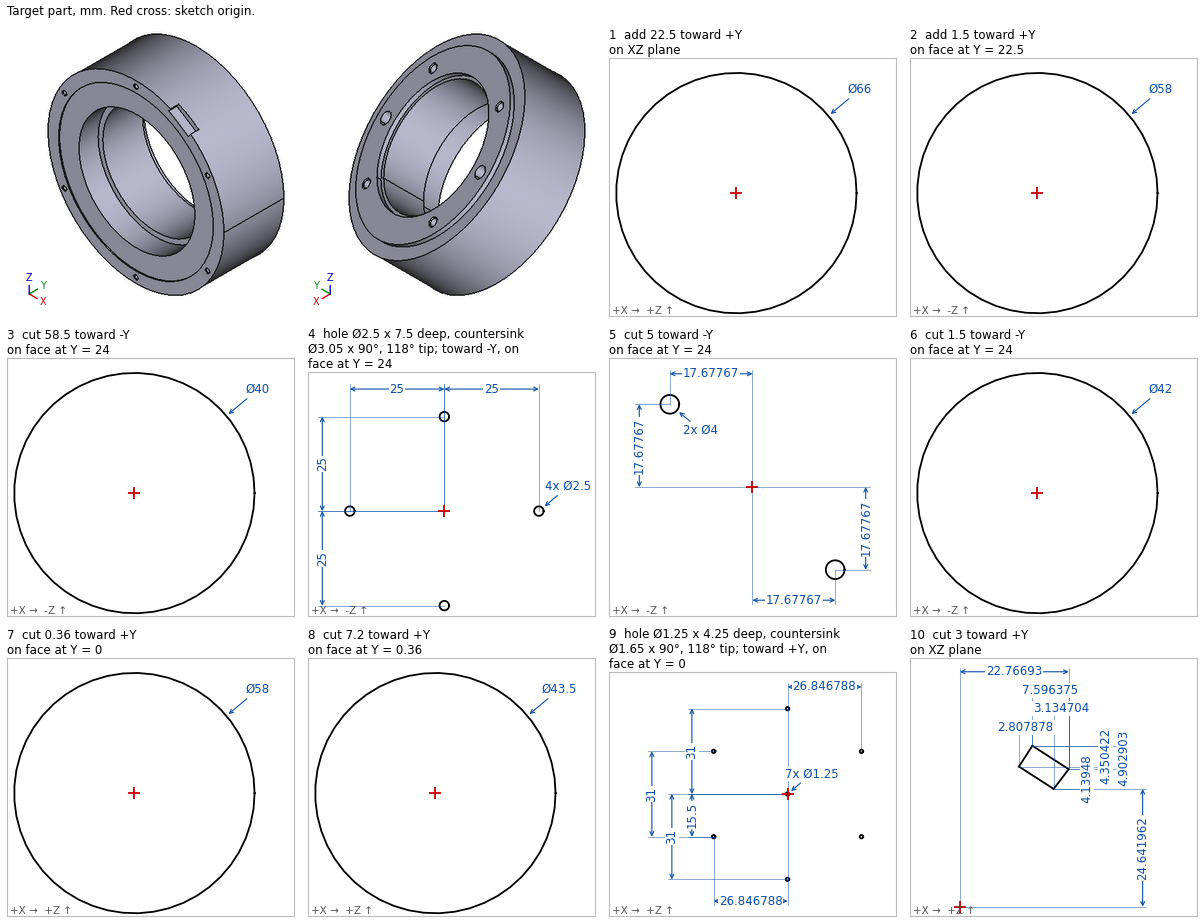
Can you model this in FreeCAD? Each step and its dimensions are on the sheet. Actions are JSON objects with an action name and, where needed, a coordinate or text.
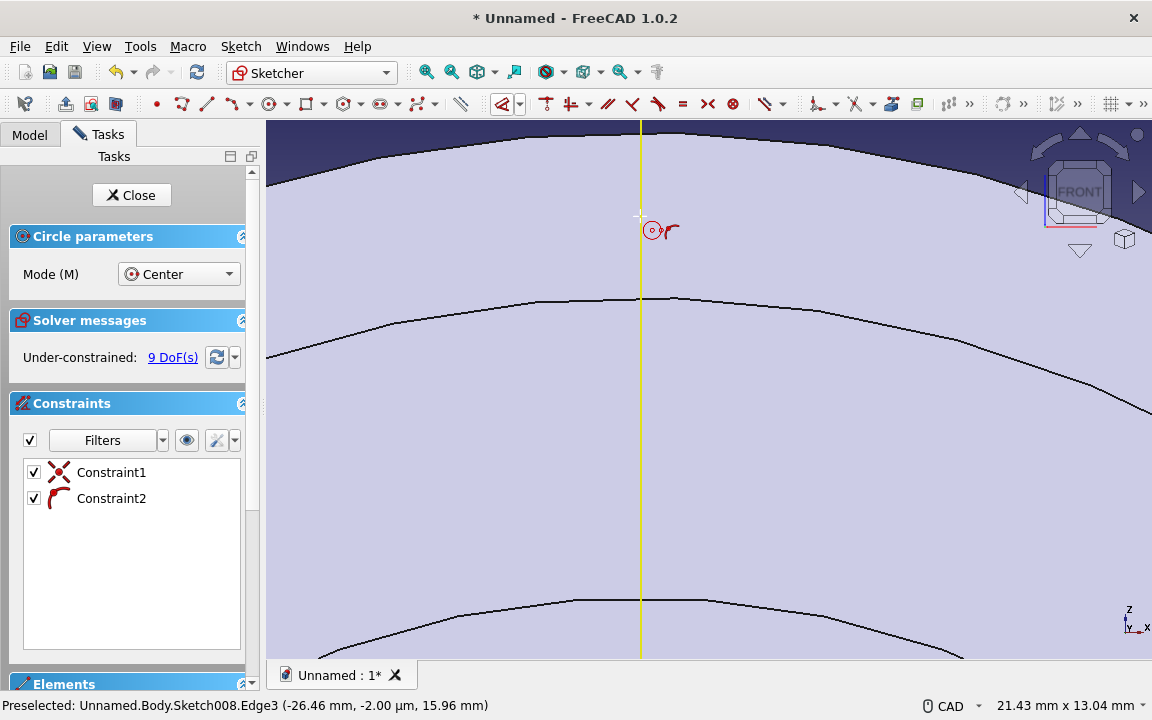
{"action": "scroll", "coordinate": [640, 216], "scroll_direction": "down", "scroll_amount": 10}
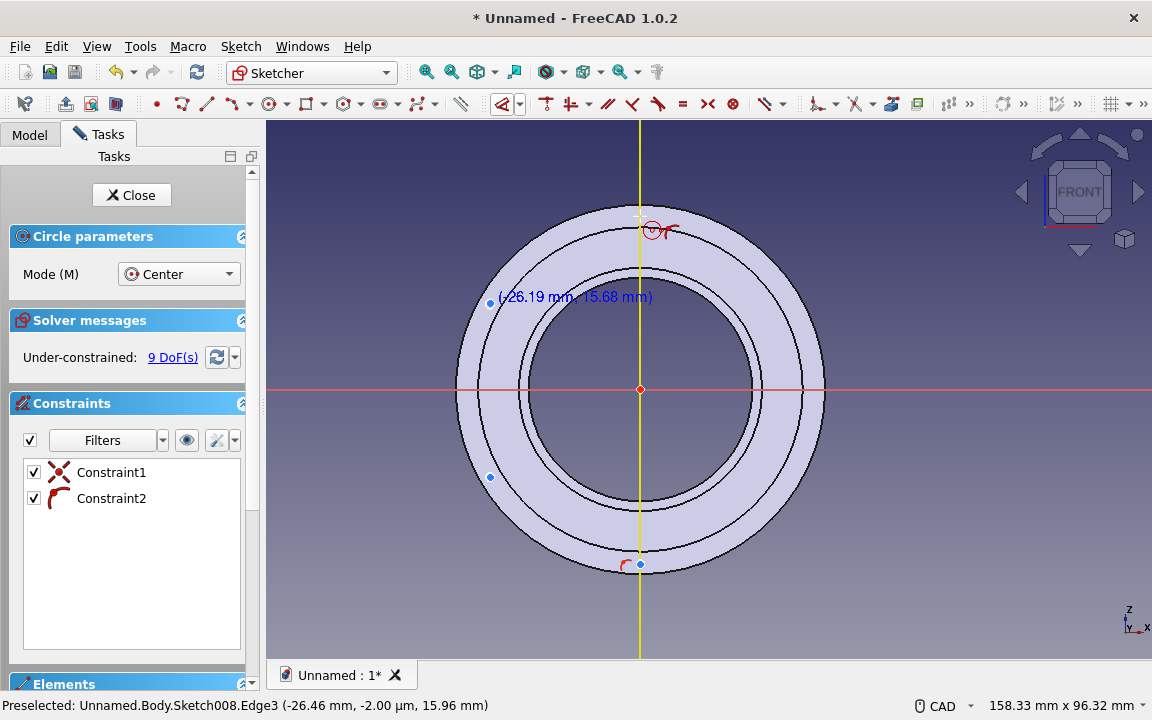
{"action": "left_click", "coordinate": [640, 216]}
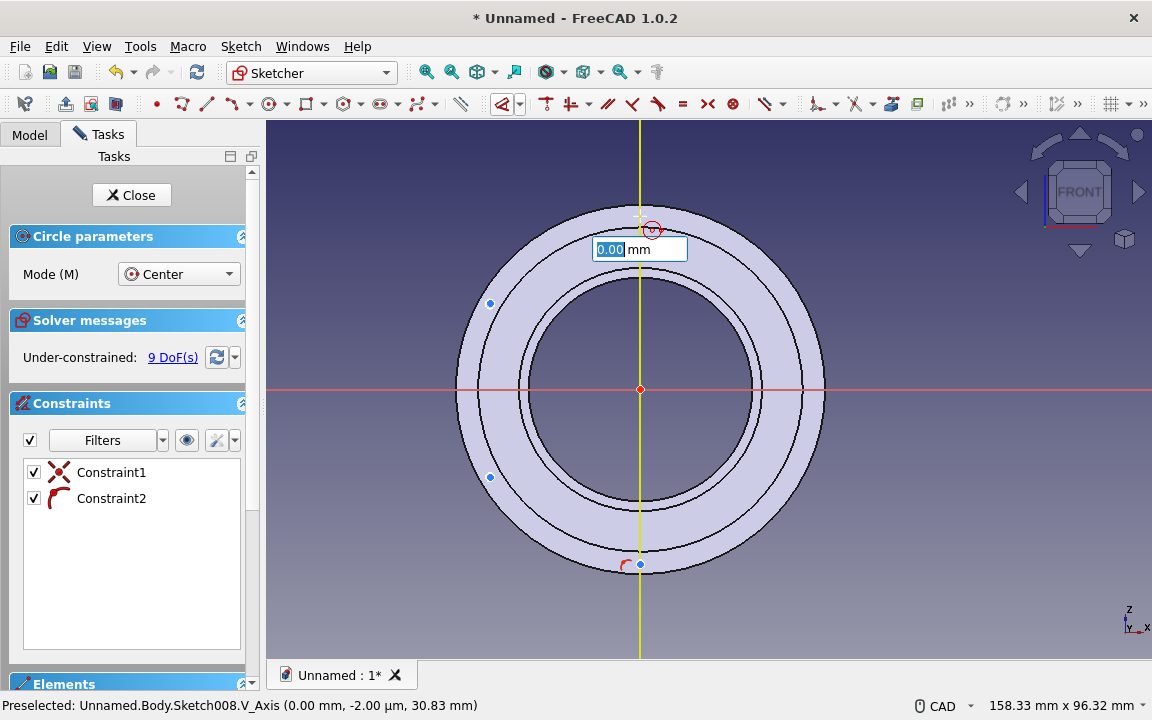
{"action": "scroll", "coordinate": [644, 215], "scroll_direction": "up", "scroll_amount": 8}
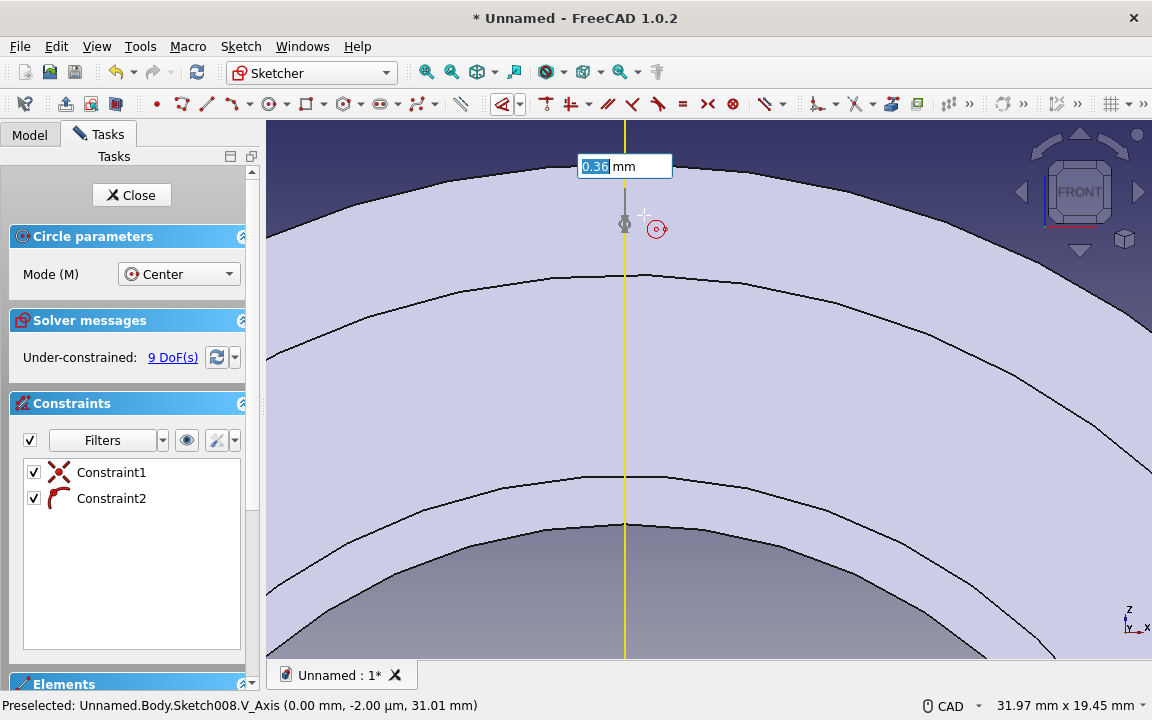
{"action": "left_click", "coordinate": [641, 213]}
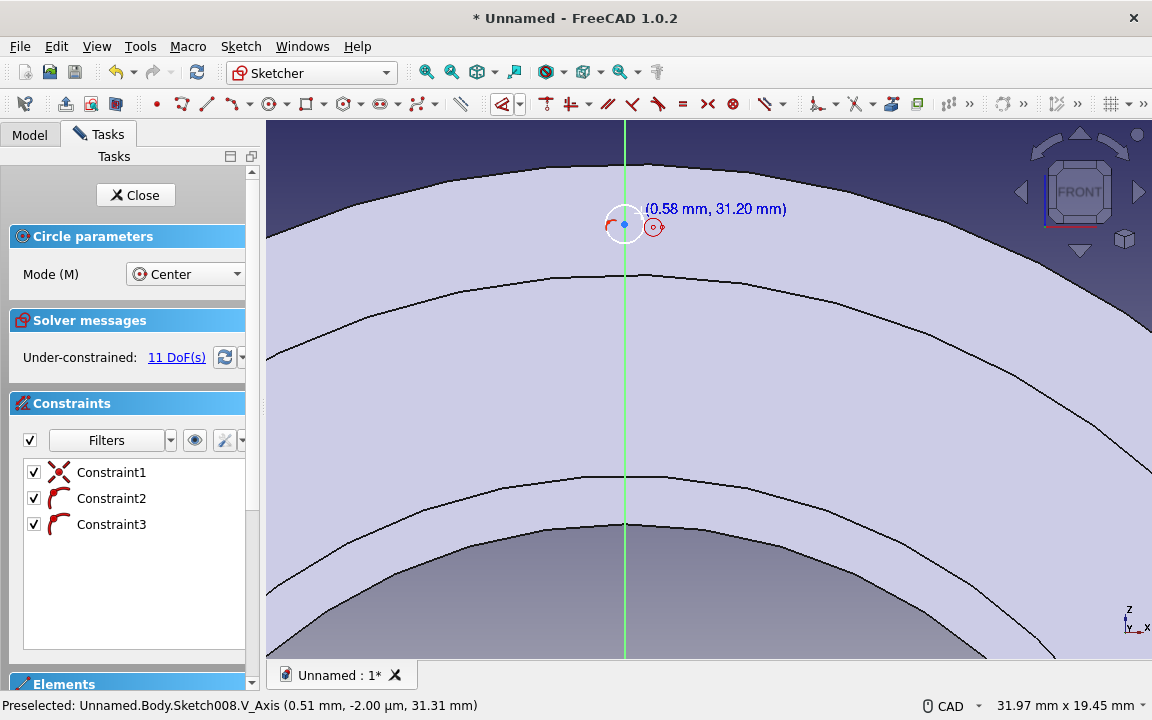
{"action": "scroll", "coordinate": [644, 215], "scroll_direction": "down", "scroll_amount": 8}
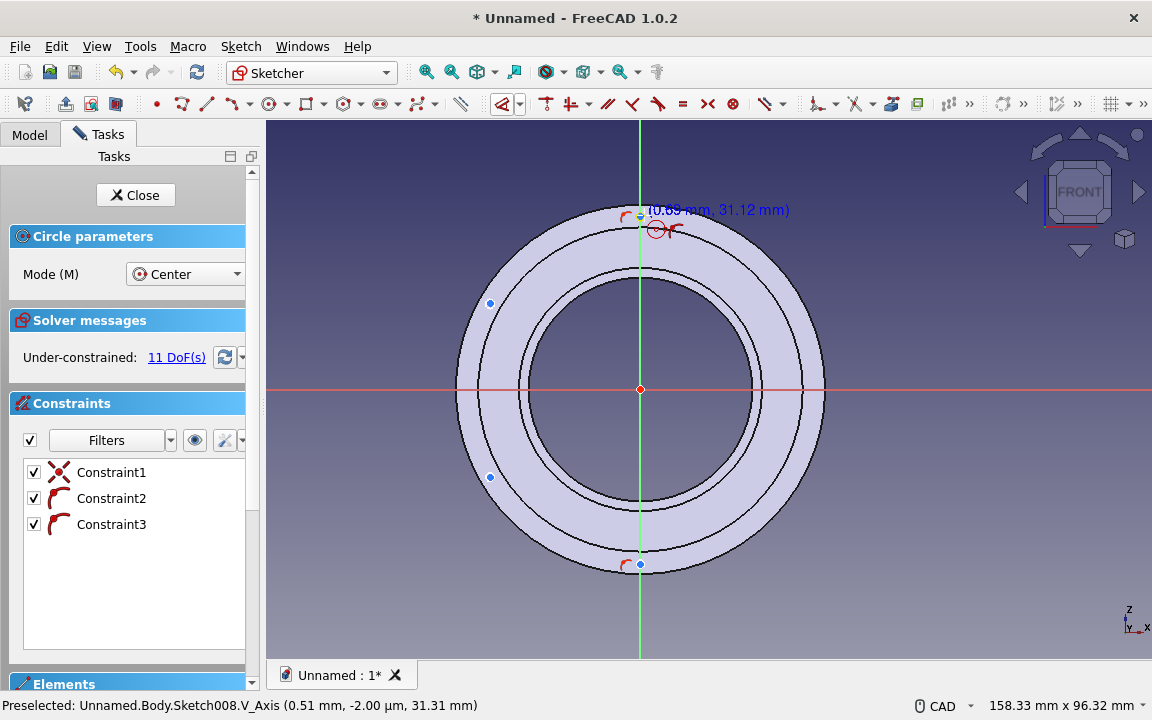
{"action": "scroll", "coordinate": [791, 303], "scroll_direction": "up", "scroll_amount": 10}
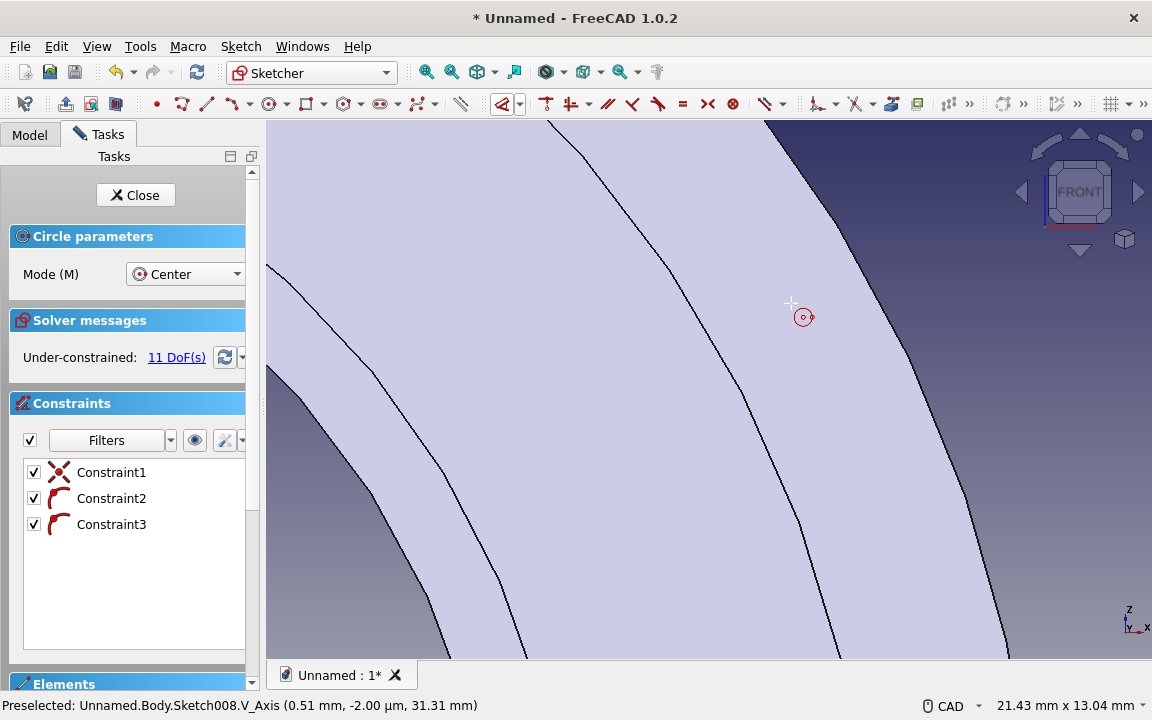
{"action": "scroll", "coordinate": [792, 303], "scroll_direction": "down", "scroll_amount": 10}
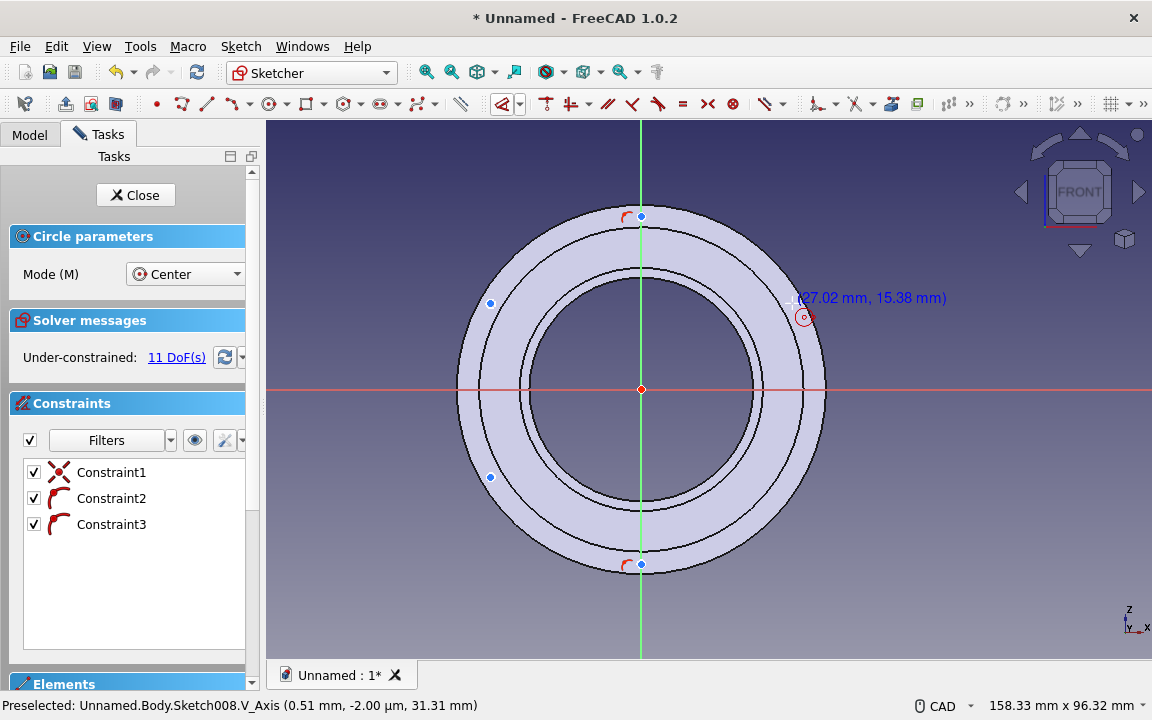
{"action": "left_click", "coordinate": [792, 303]}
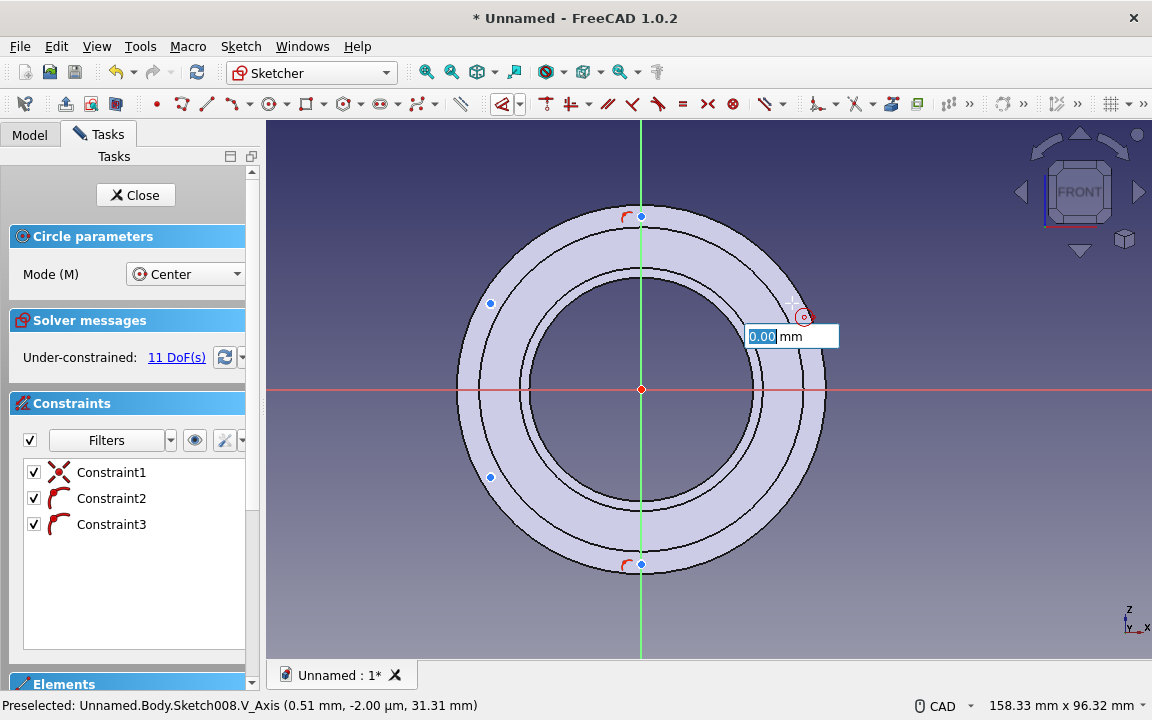
{"action": "scroll", "coordinate": [794, 300], "scroll_direction": "up", "scroll_amount": 8}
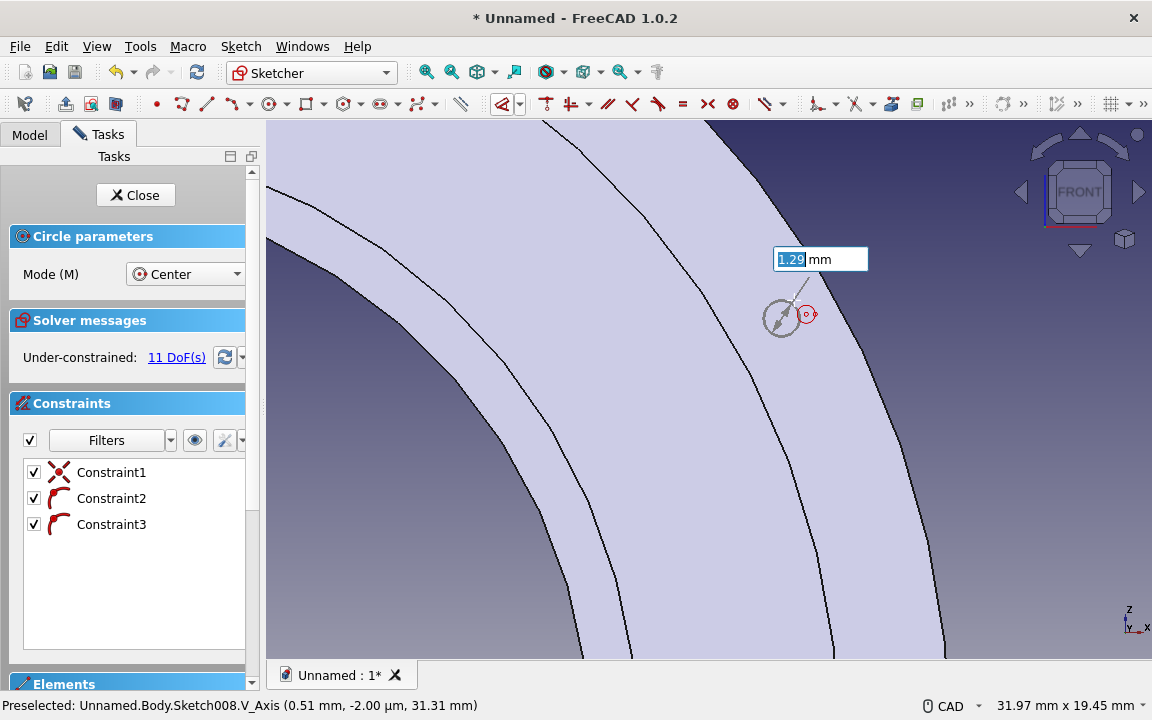
{"action": "left_click", "coordinate": [792, 300]}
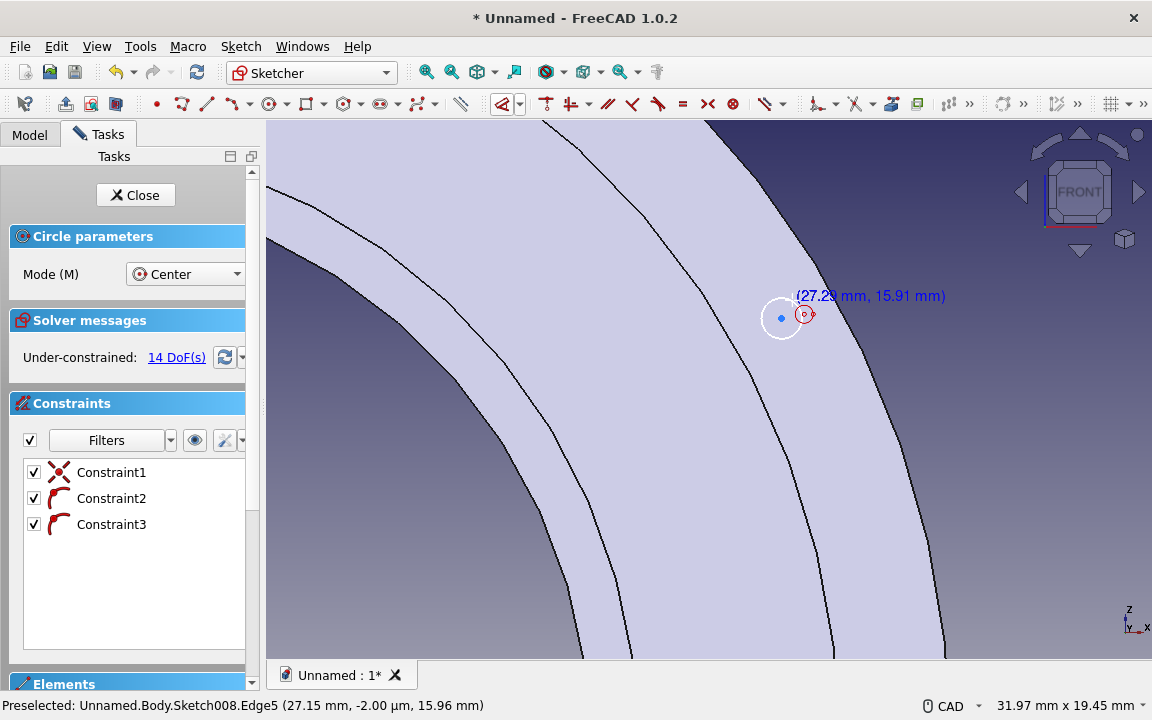
{"action": "scroll", "coordinate": [794, 300], "scroll_direction": "down", "scroll_amount": 8}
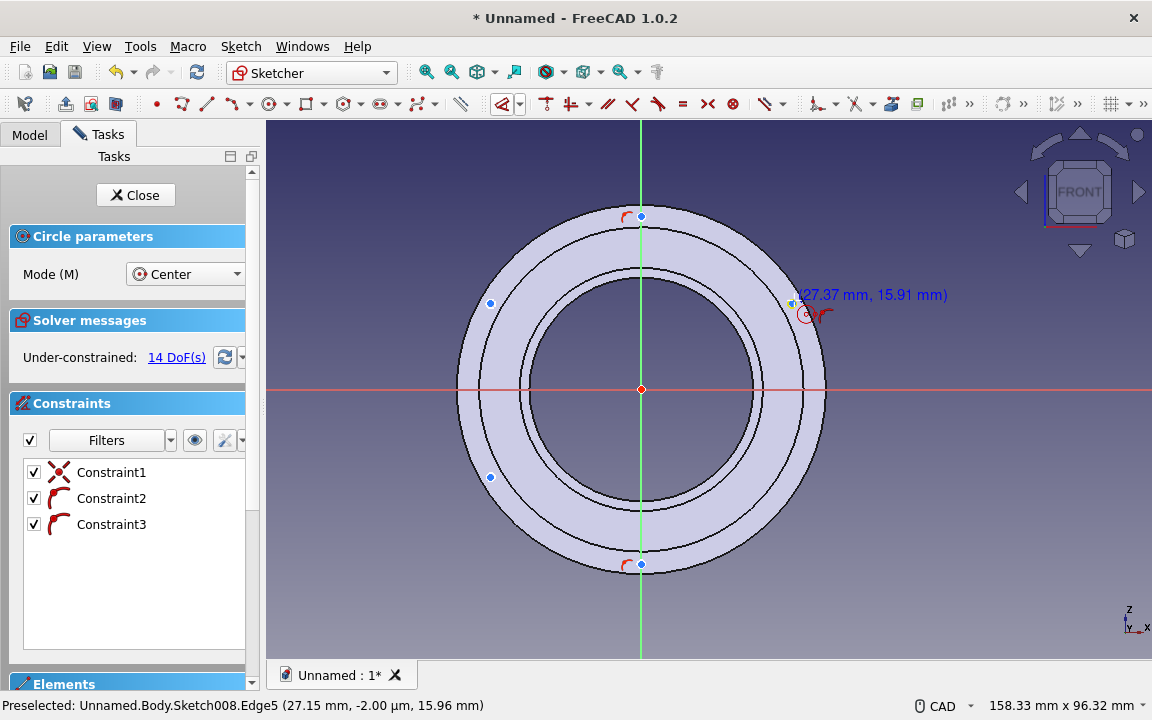
{"action": "scroll", "coordinate": [792, 476], "scroll_direction": "up", "scroll_amount": 10}